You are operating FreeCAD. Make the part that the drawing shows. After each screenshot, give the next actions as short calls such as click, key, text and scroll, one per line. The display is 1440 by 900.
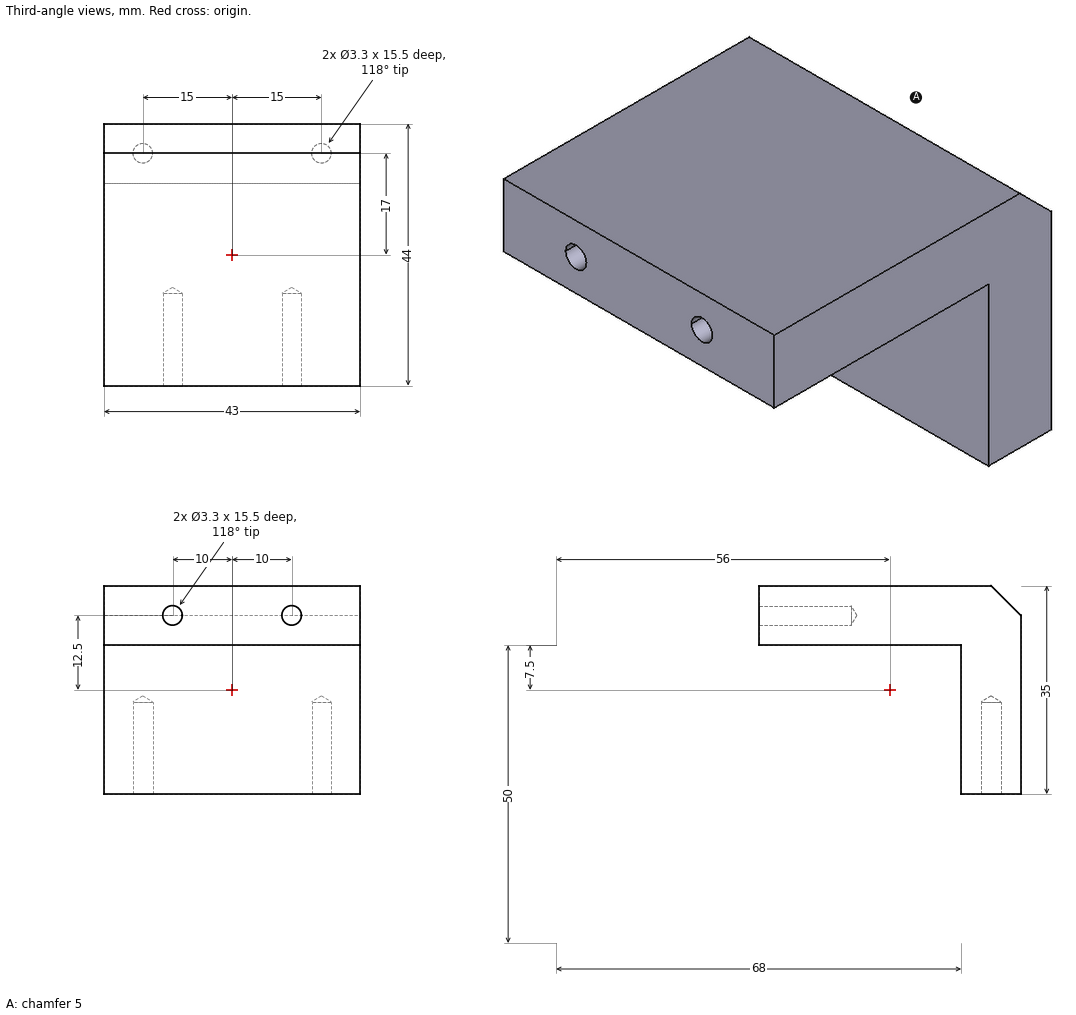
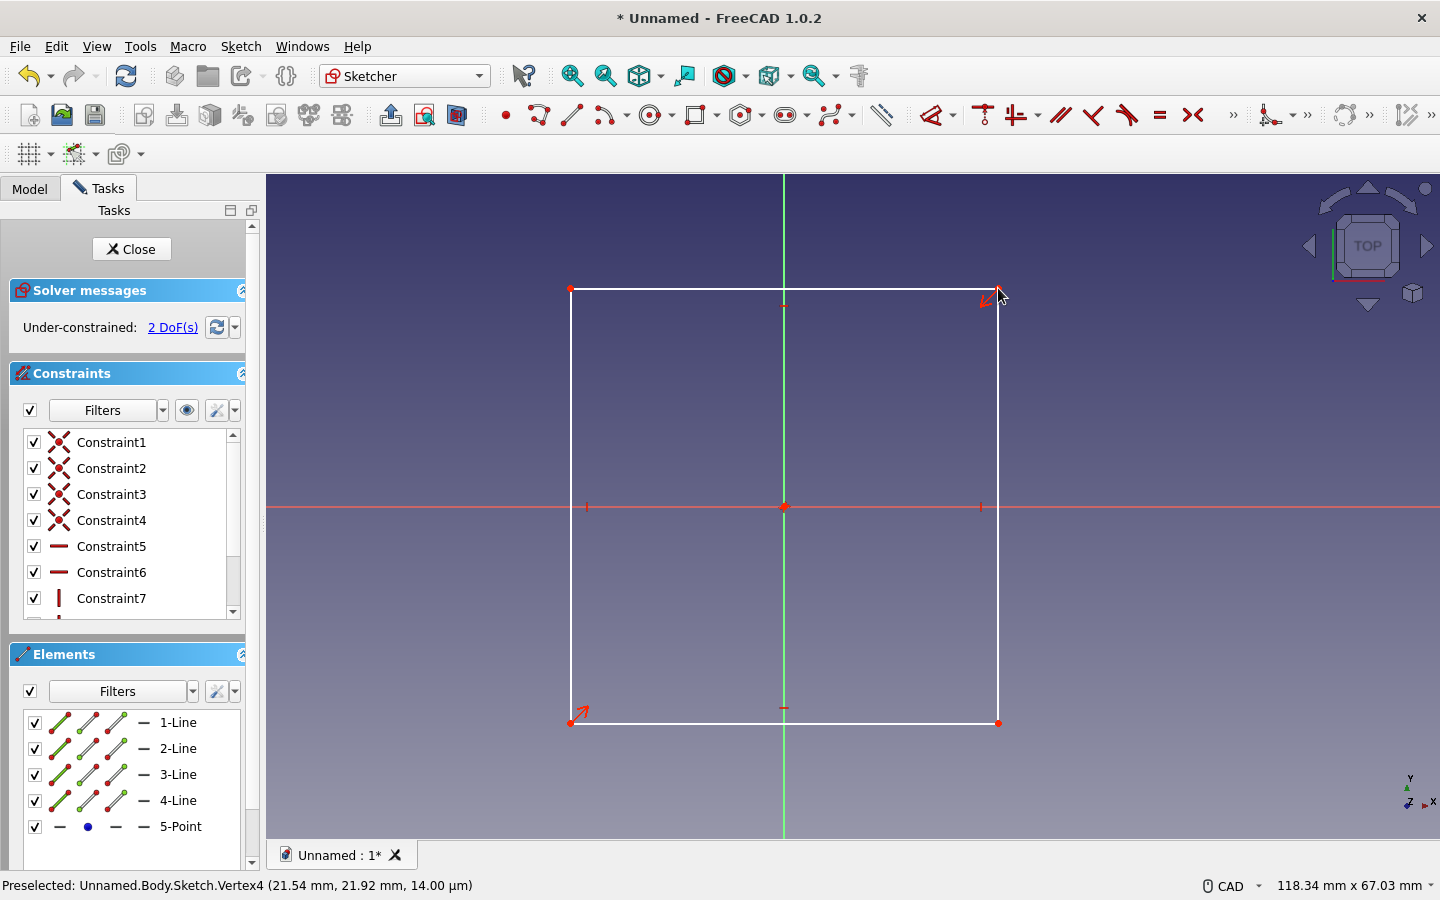
click(930, 116)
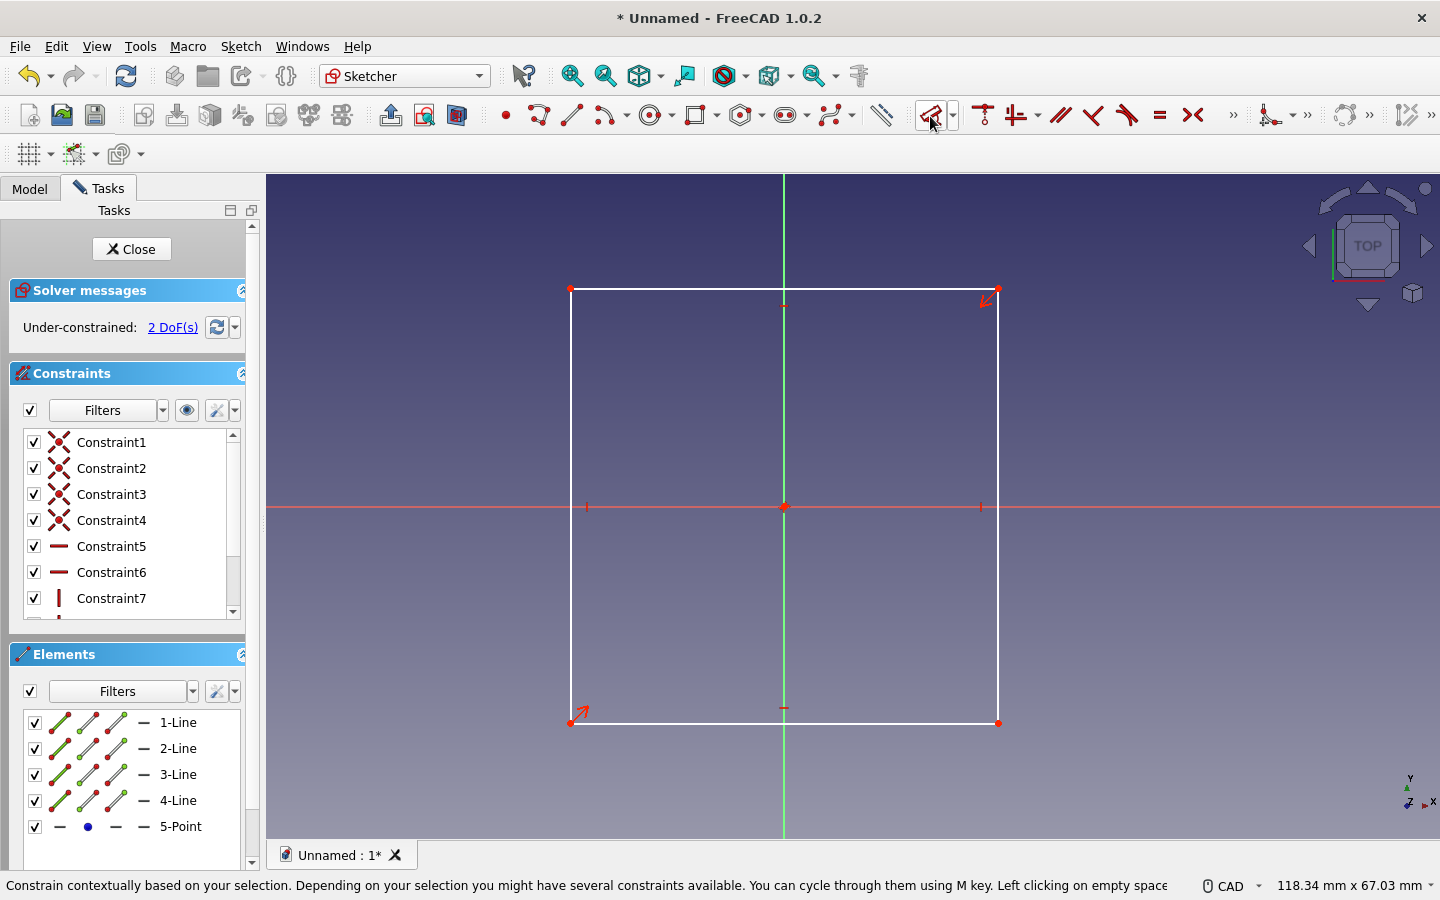
click(699, 724)
click(686, 758)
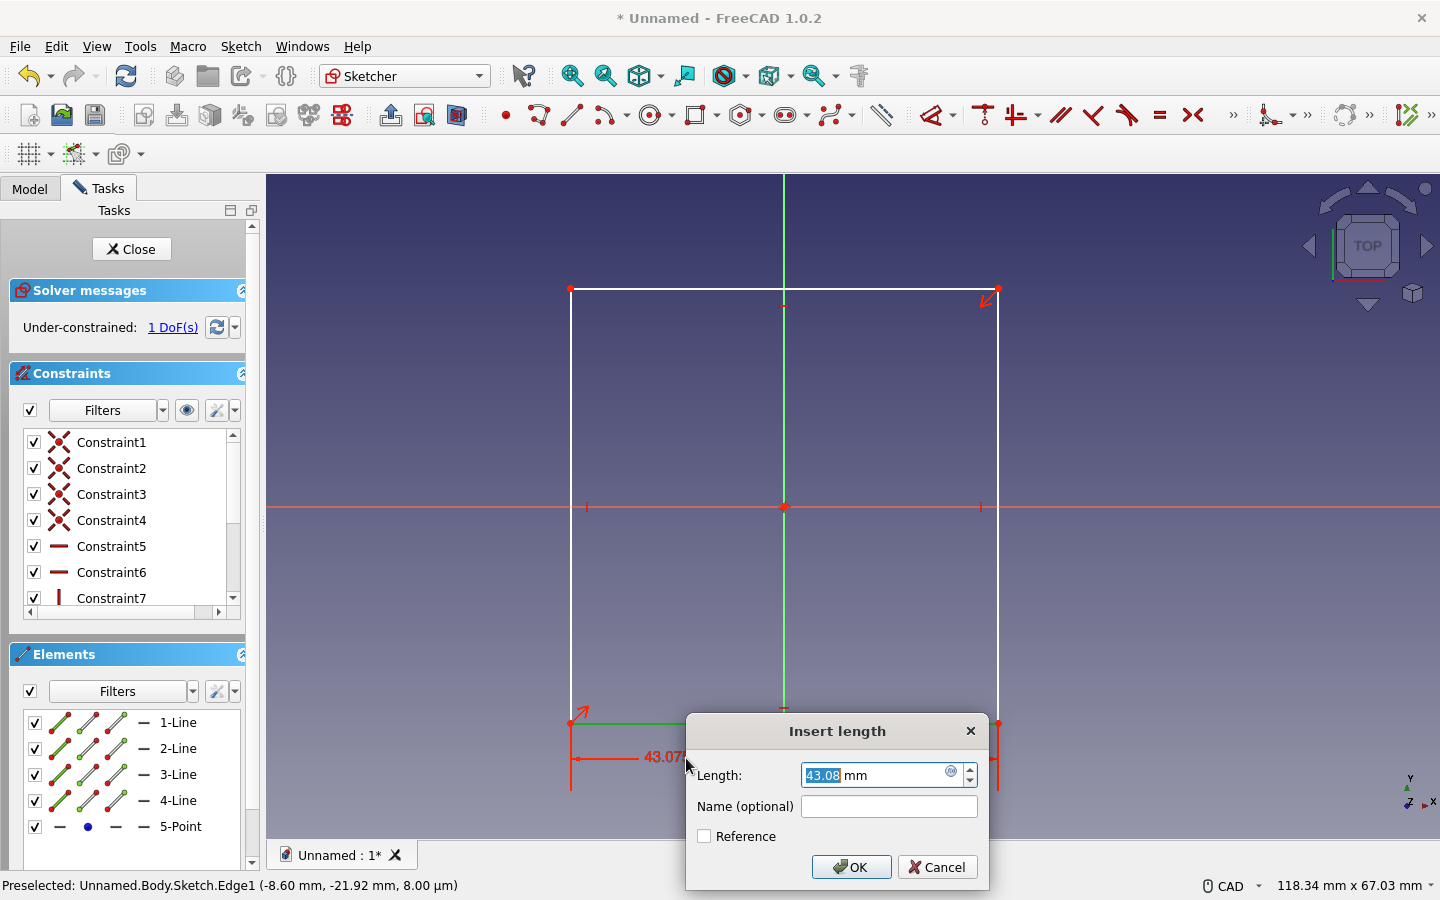
text(43)
key(Return)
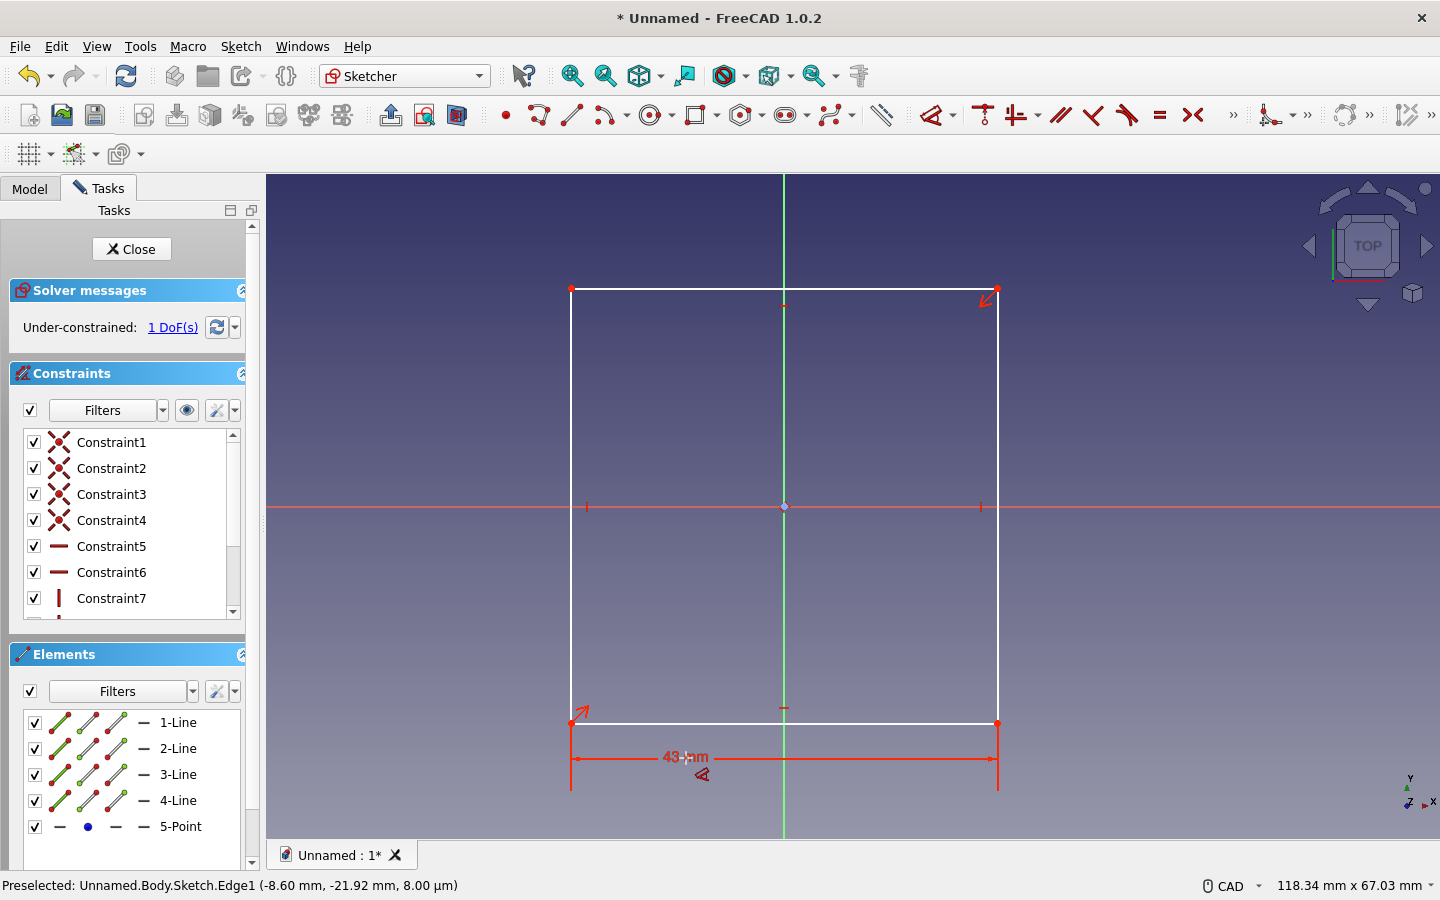
click(998, 594)
click(1032, 406)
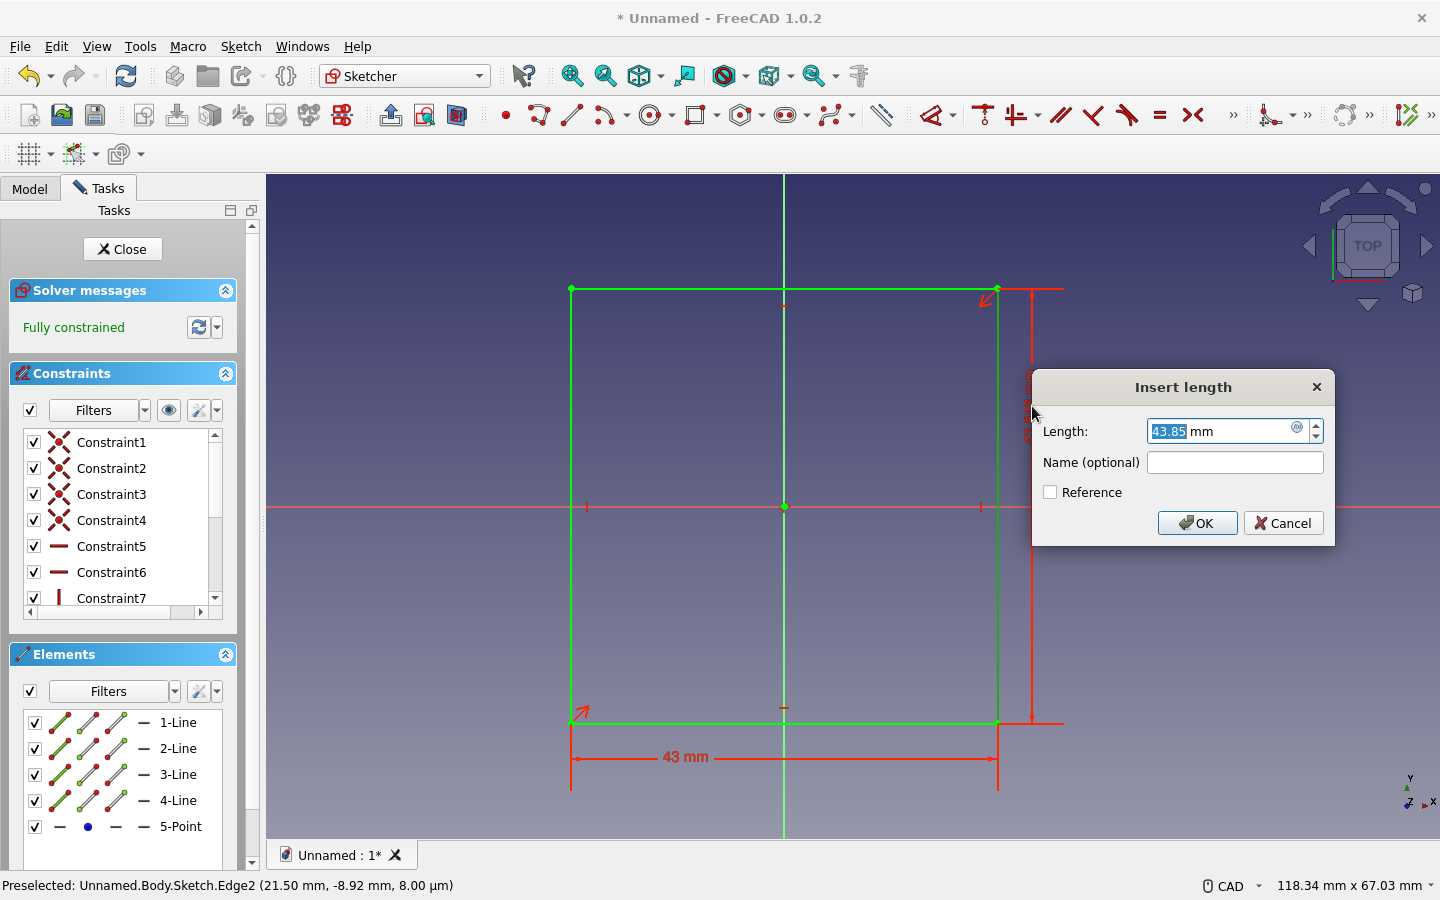
text(44)
key(Return)
key(Escape)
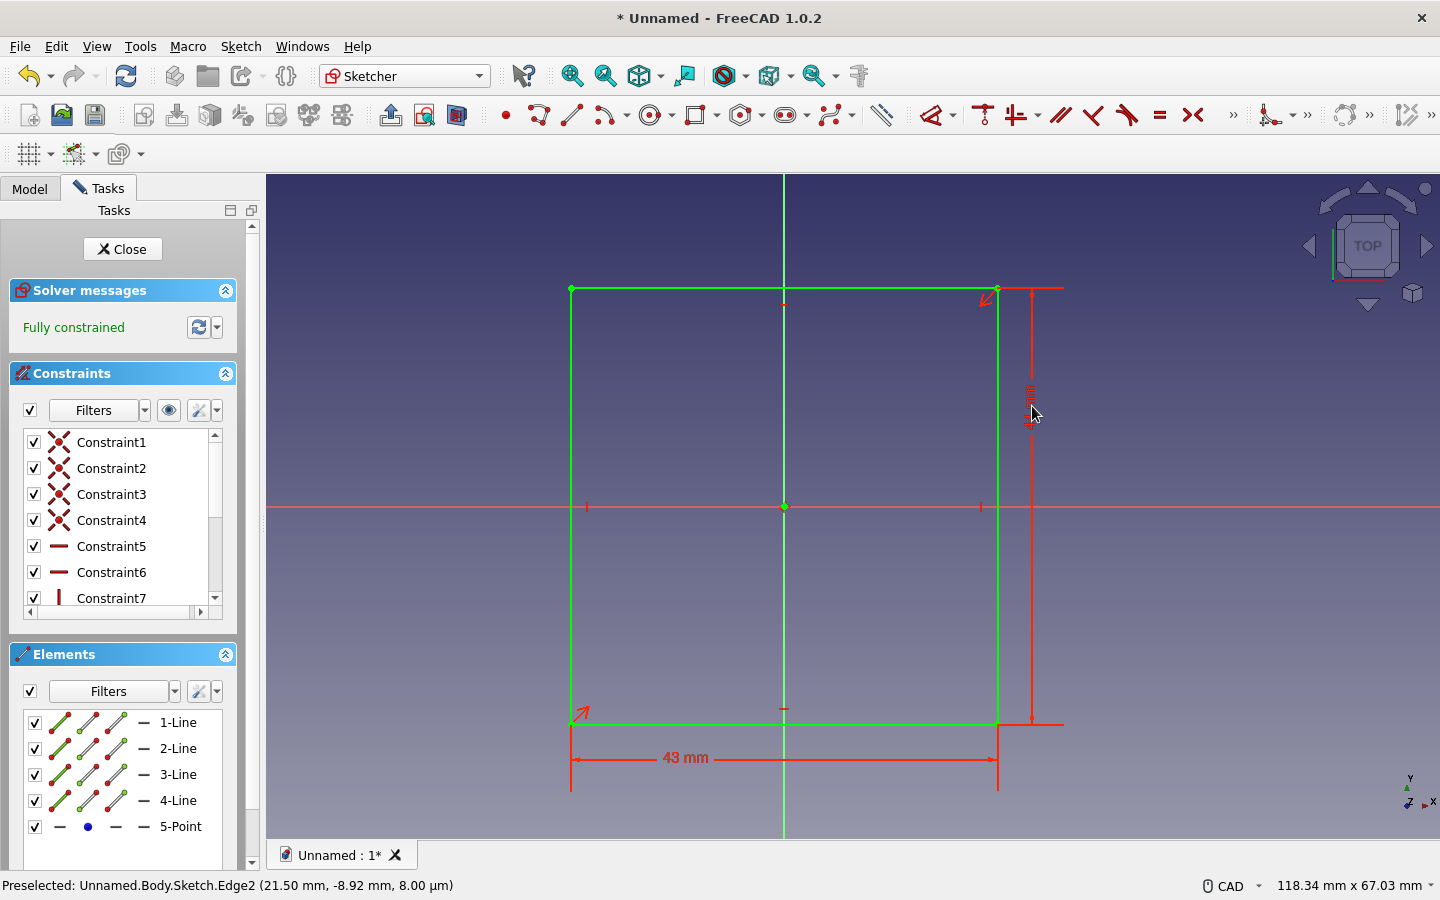
click(123, 249)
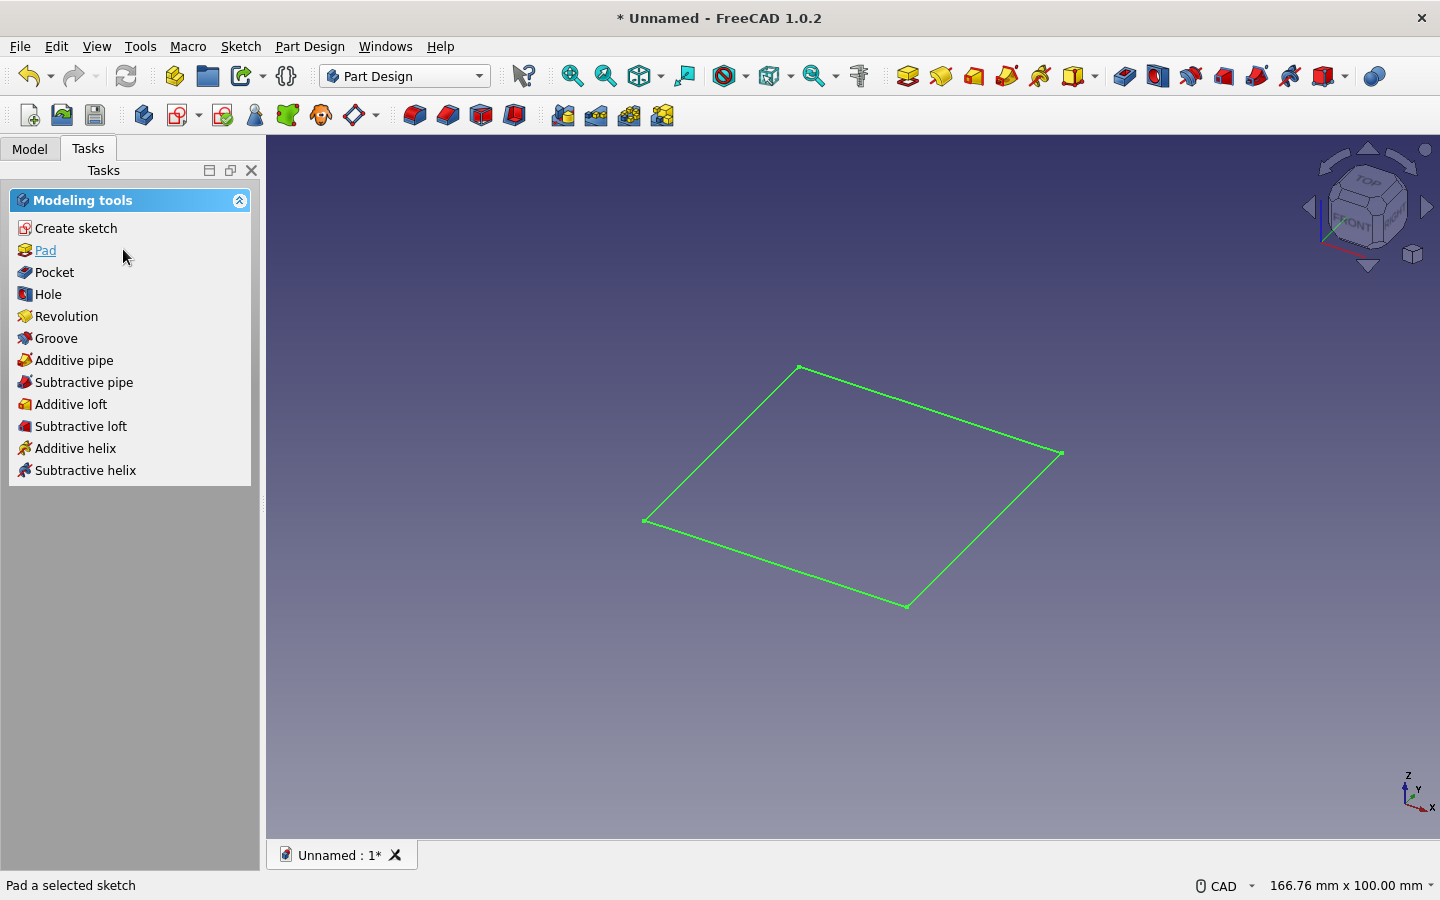
click(908, 76)